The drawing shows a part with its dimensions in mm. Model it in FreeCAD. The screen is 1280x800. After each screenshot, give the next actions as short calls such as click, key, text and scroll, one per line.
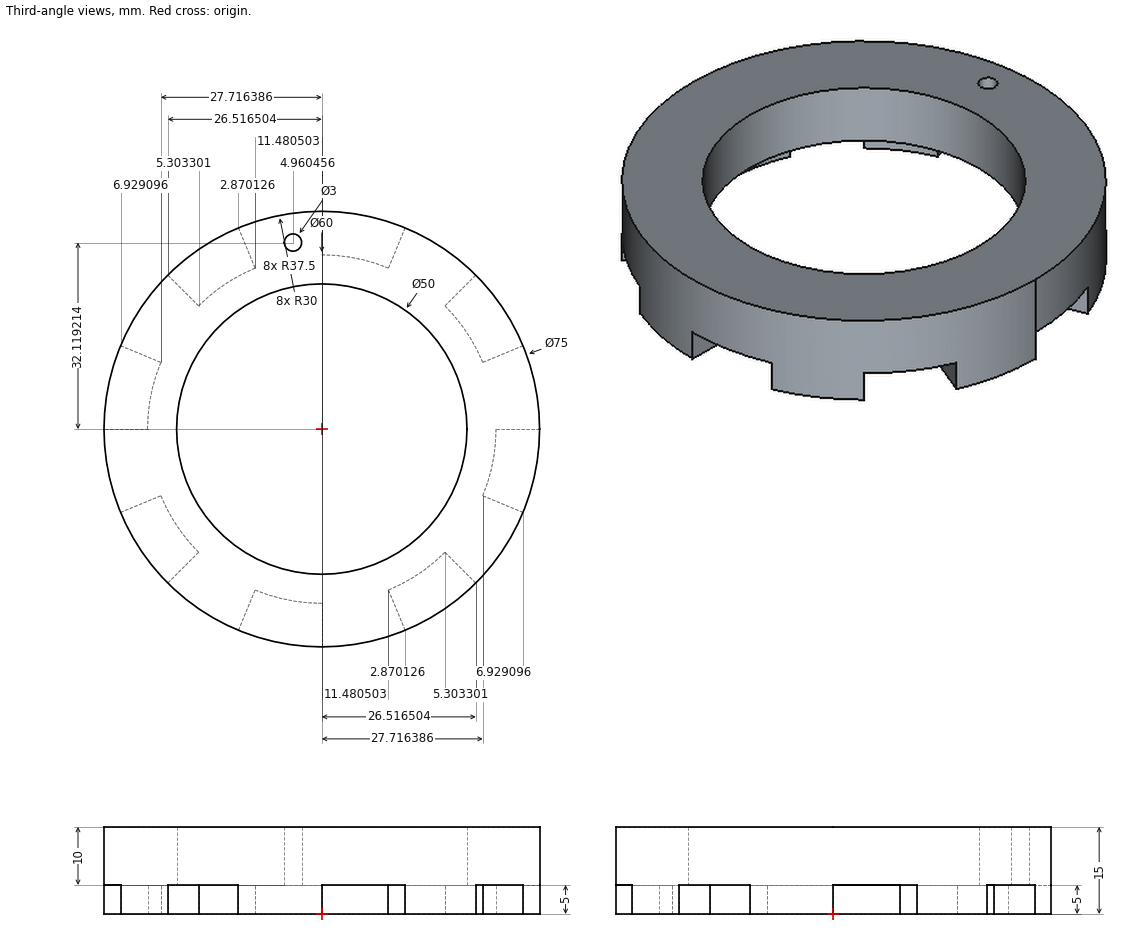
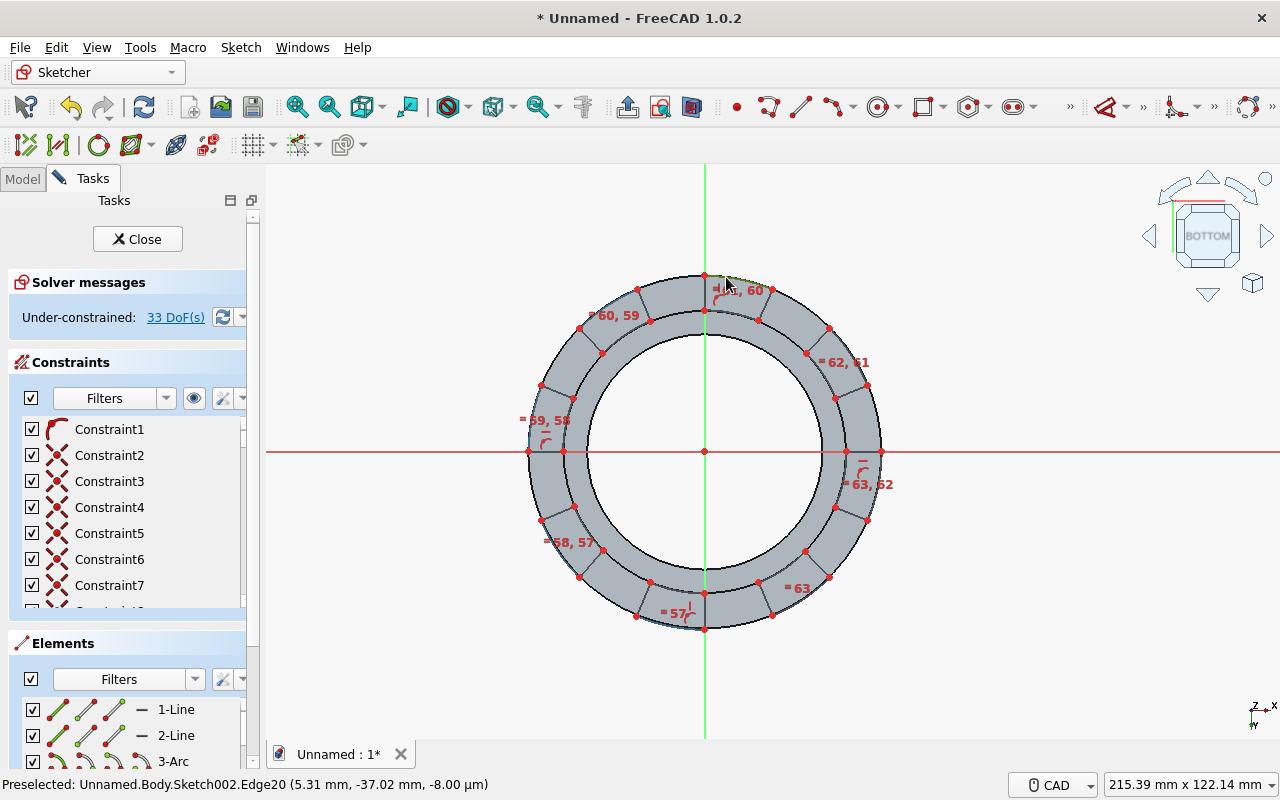
click(843, 344)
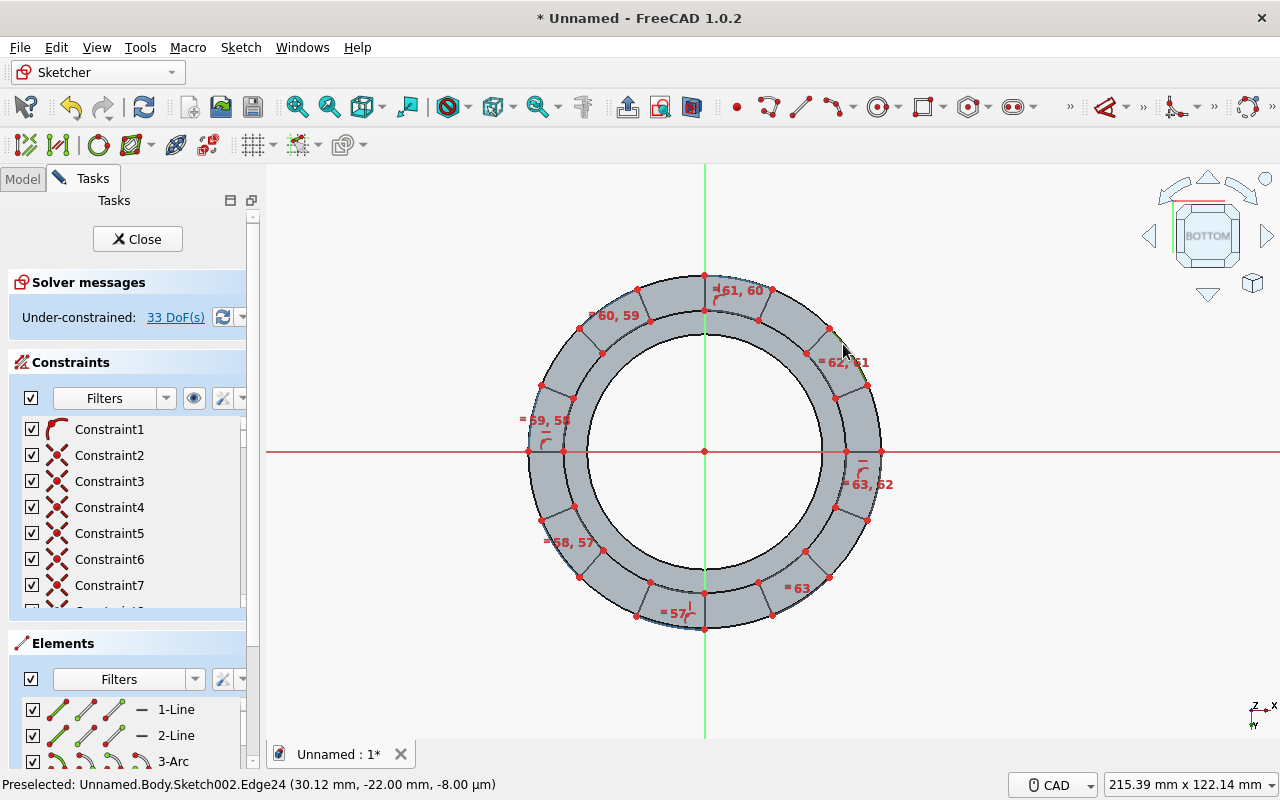
click(875, 501)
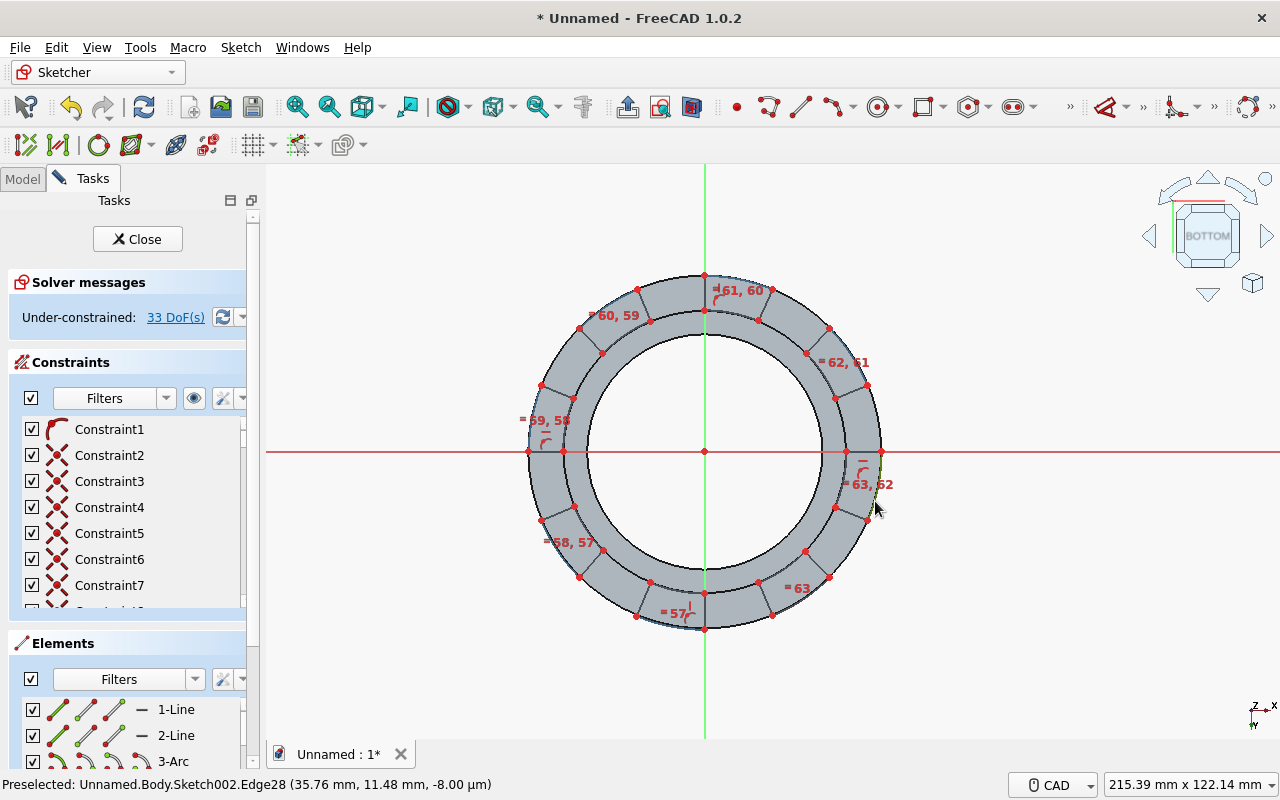
click(791, 607)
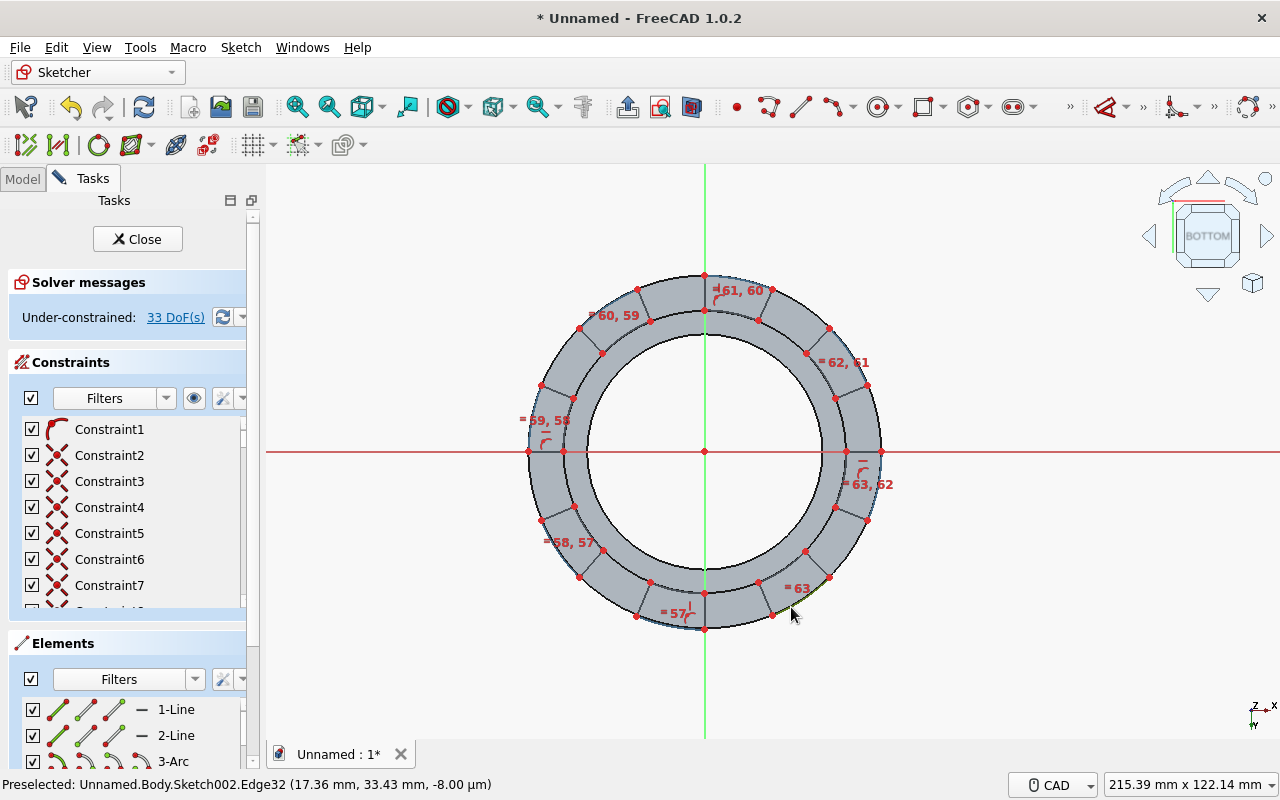
key(e)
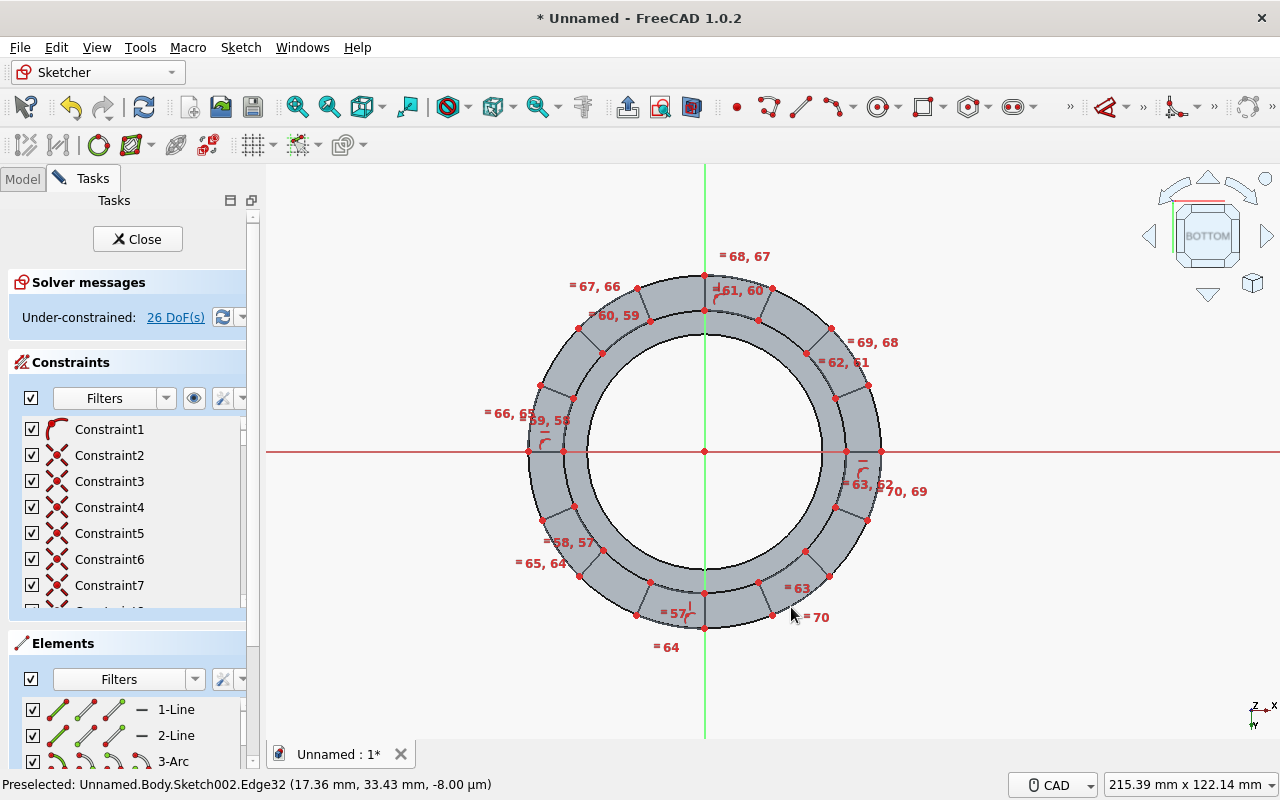
key(d)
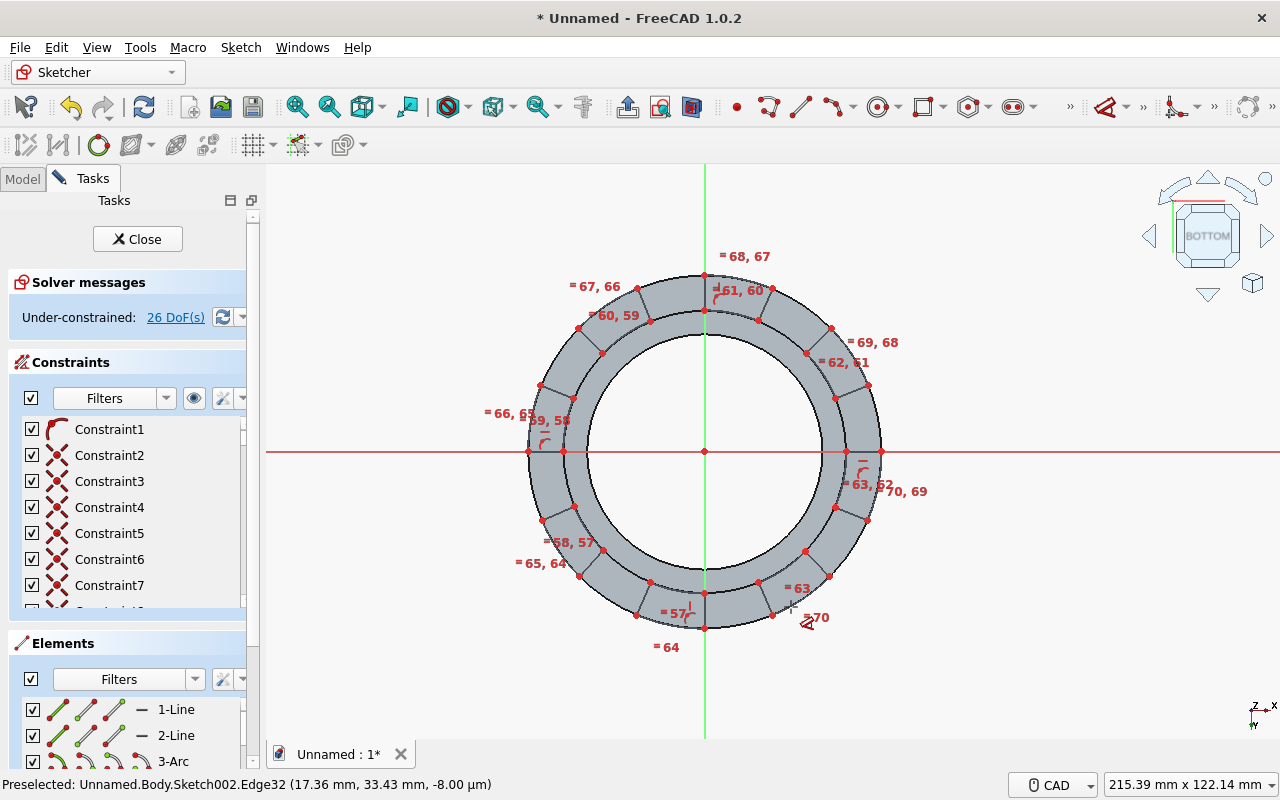
click(666, 588)
click(743, 621)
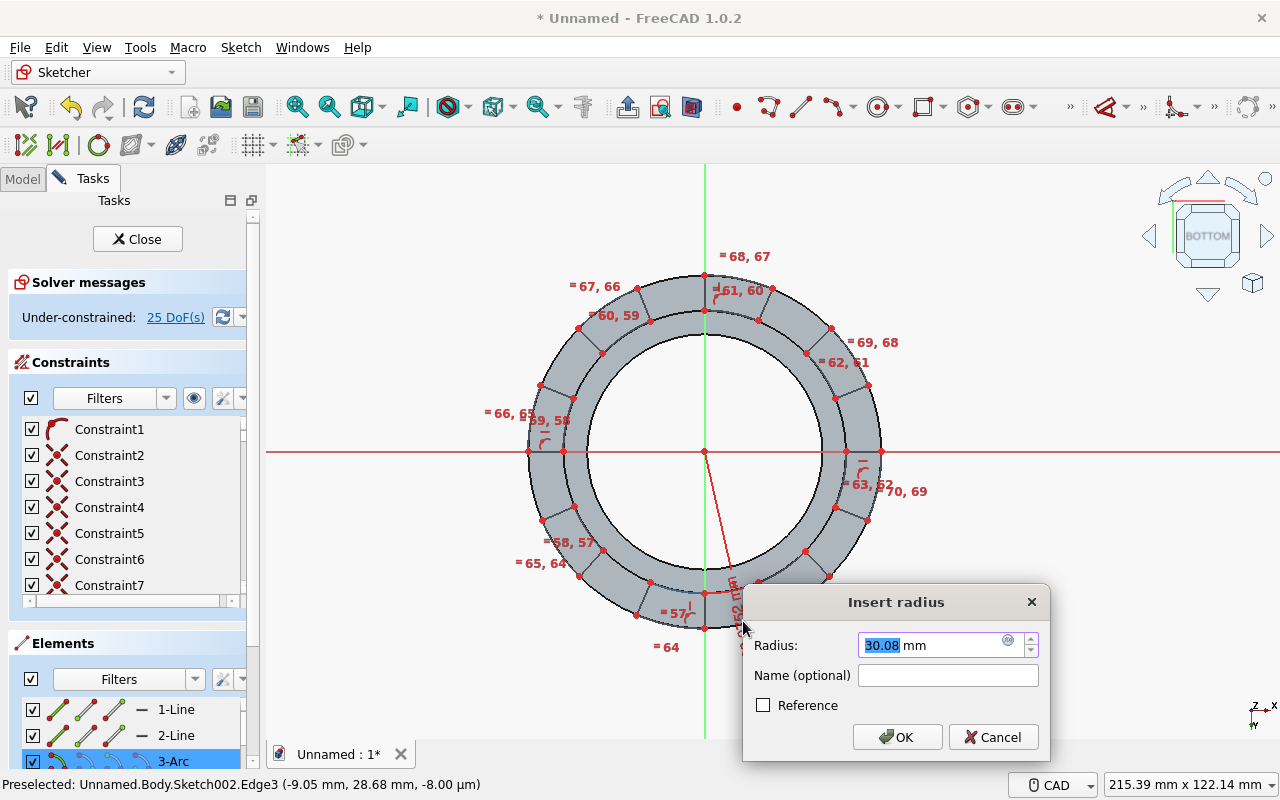
text(30)
key(Return)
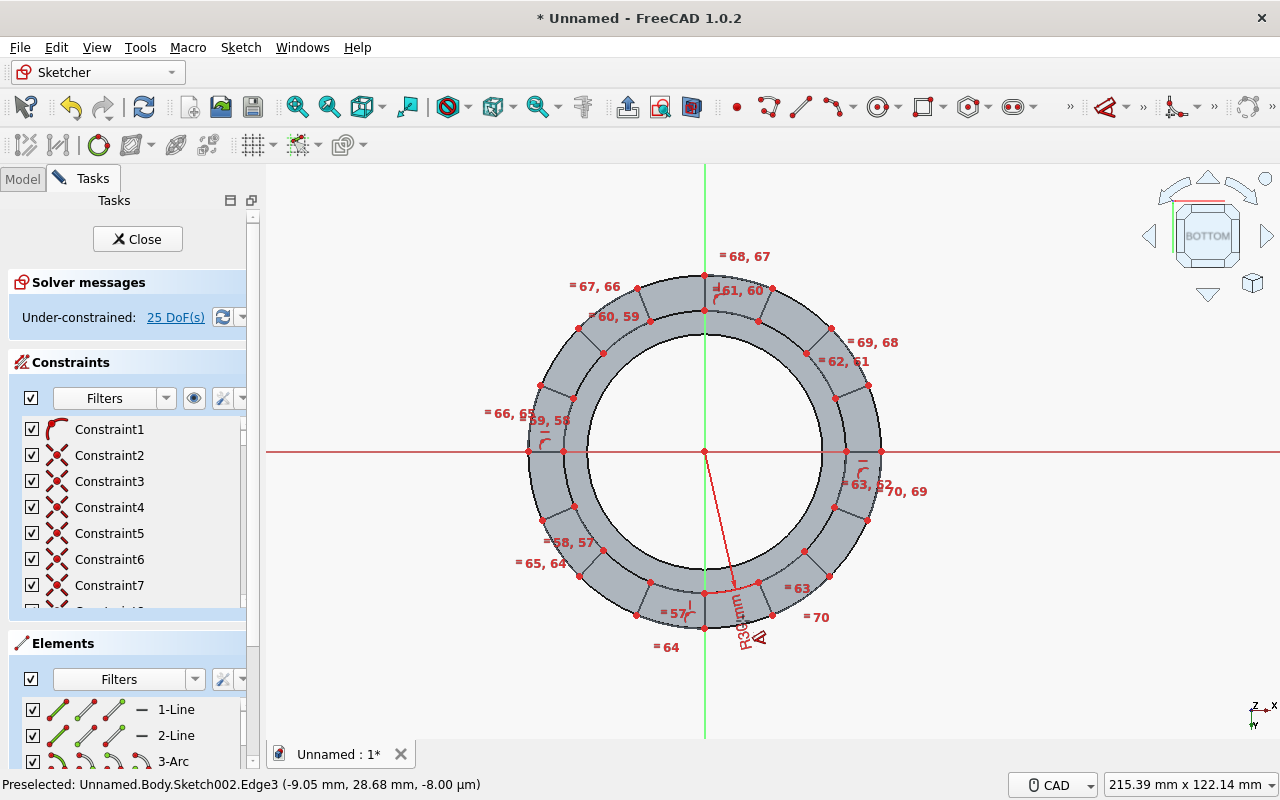
click(657, 622)
click(648, 653)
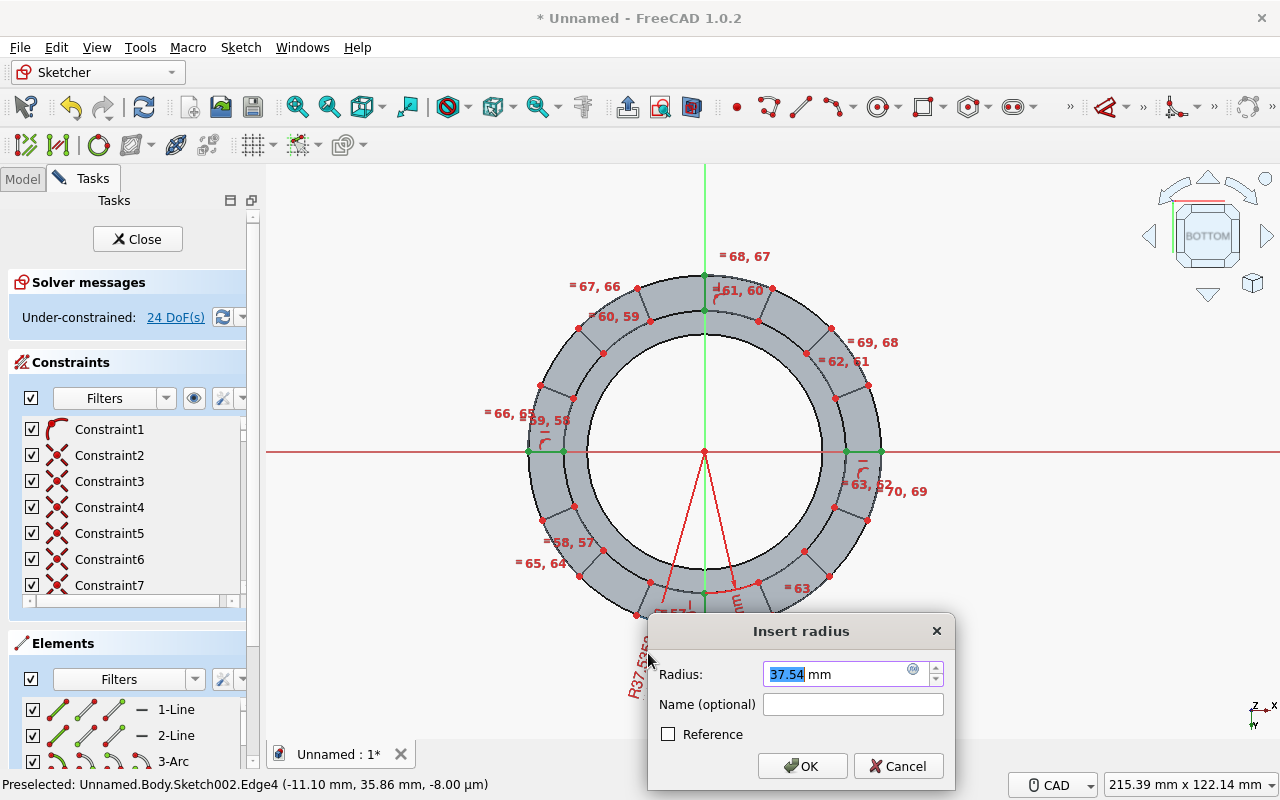
text(37.5)
key(Return)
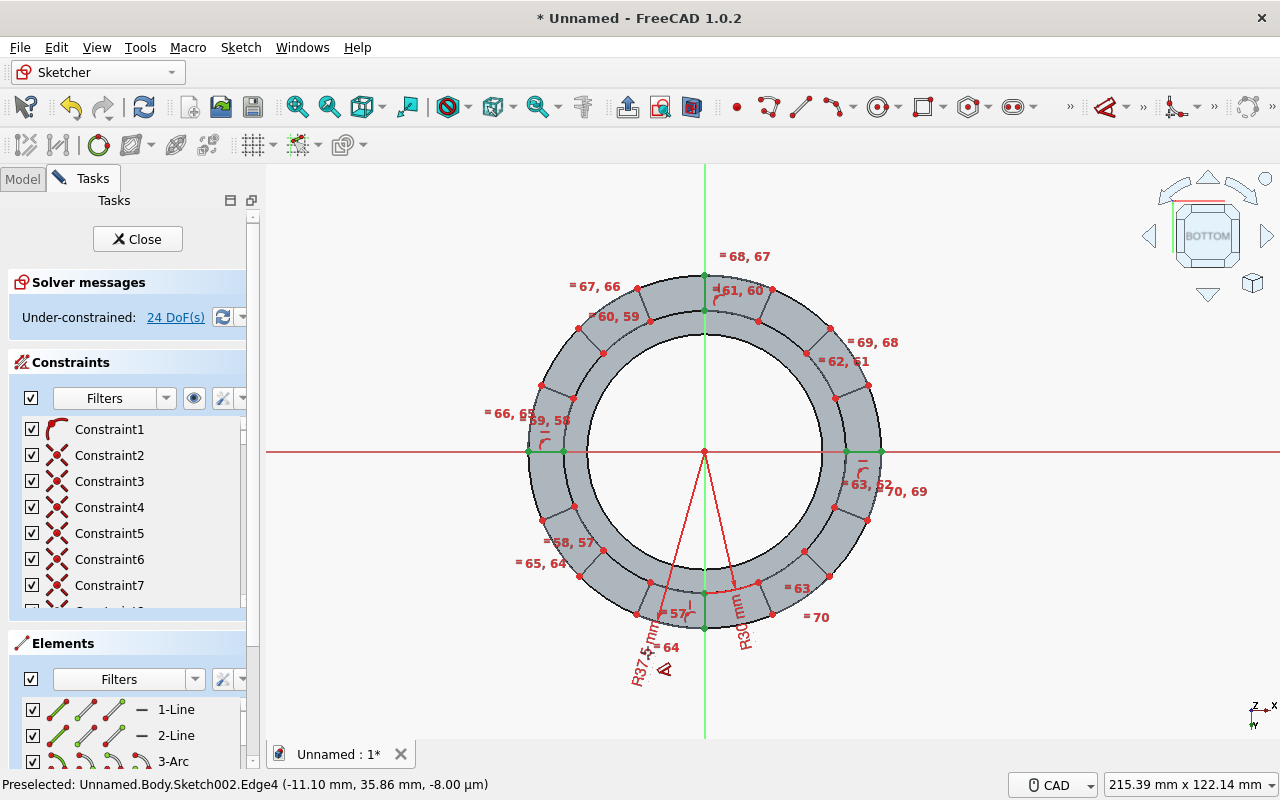
scroll(647, 592, up, 6)